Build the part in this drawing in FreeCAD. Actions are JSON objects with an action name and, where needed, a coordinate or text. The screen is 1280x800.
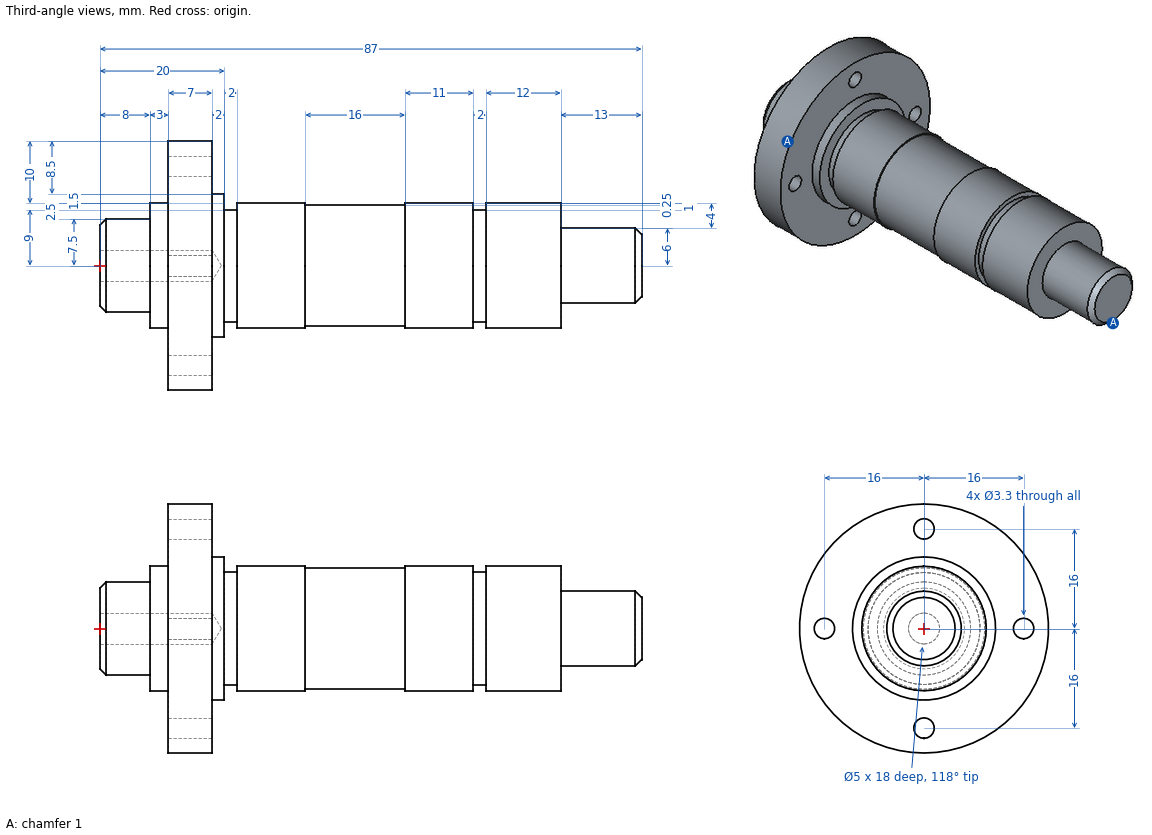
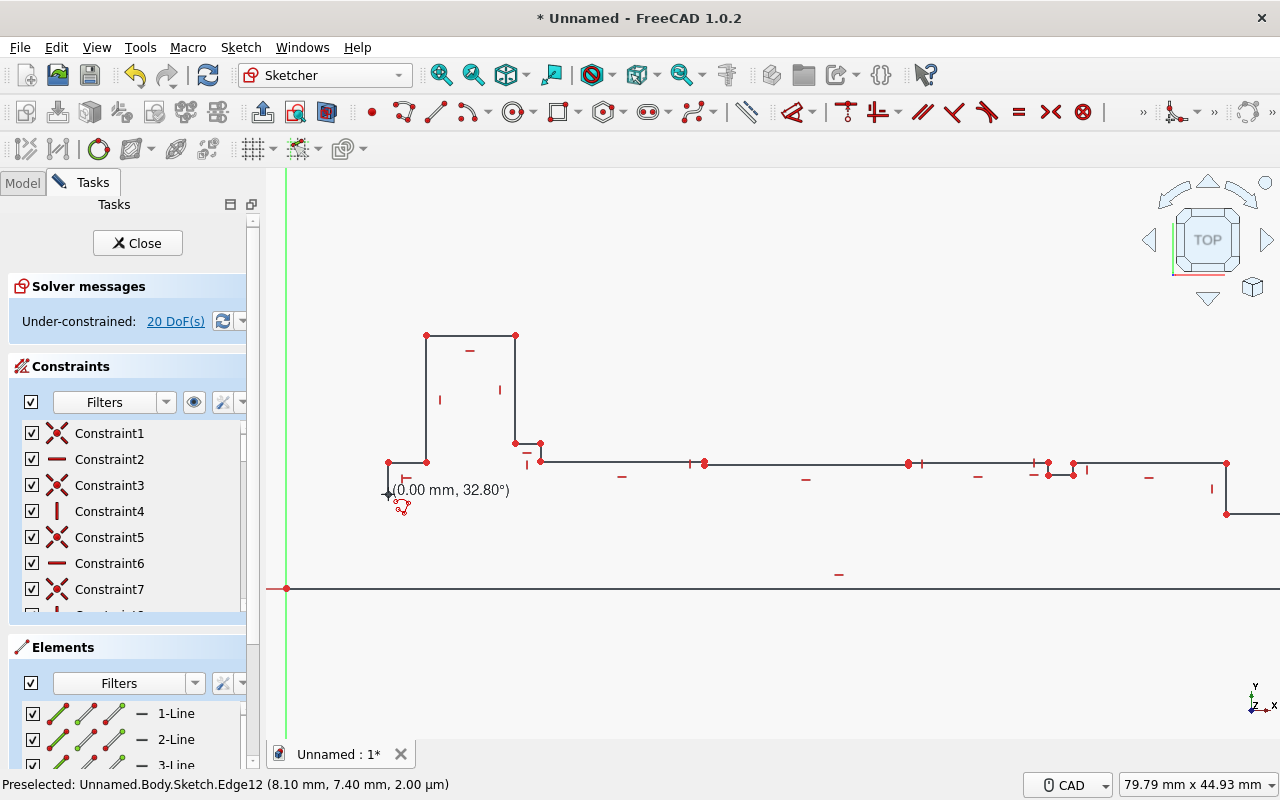
{"action": "scroll", "coordinate": [541, 443], "scroll_direction": "down", "scroll_amount": 3}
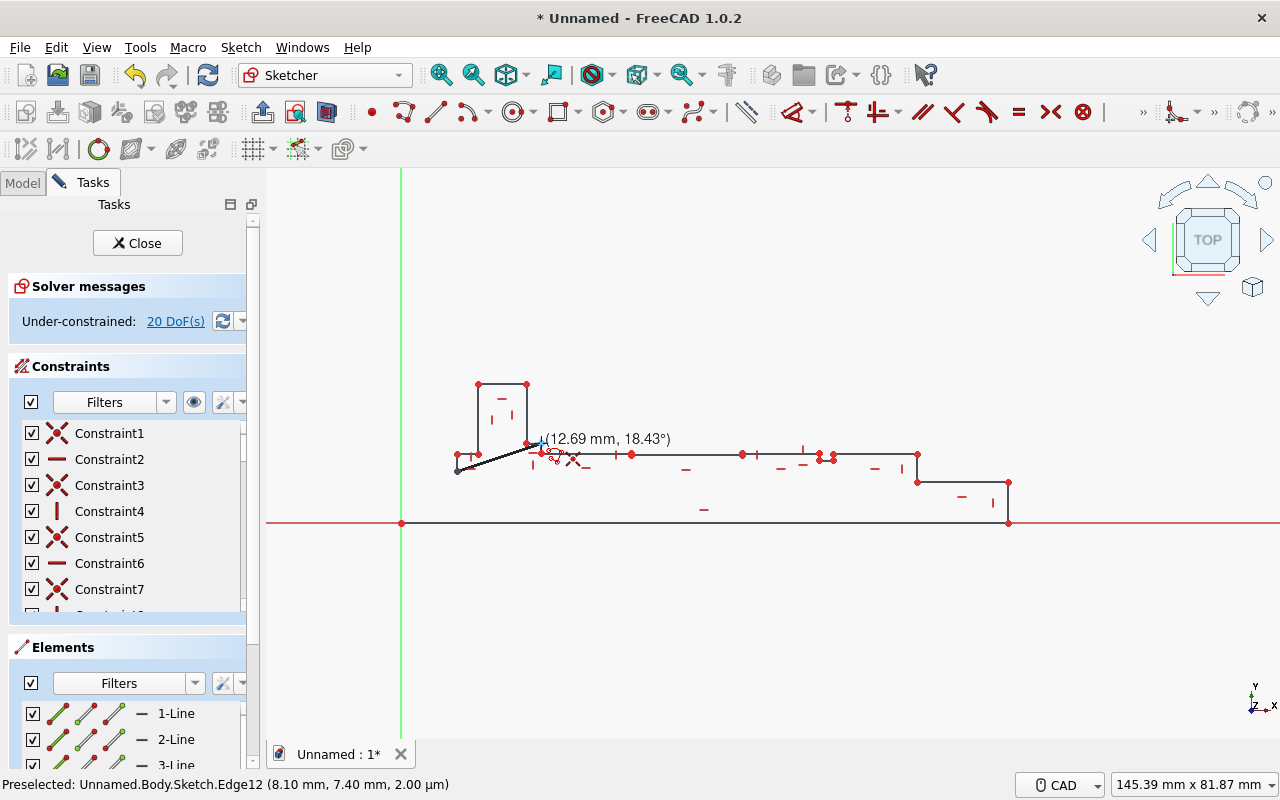
{"action": "left_click", "coordinate": [410, 471]}
{"action": "left_click", "coordinate": [401, 523]}
{"action": "key", "text": "Escape"}
{"action": "key", "text": "Escape"}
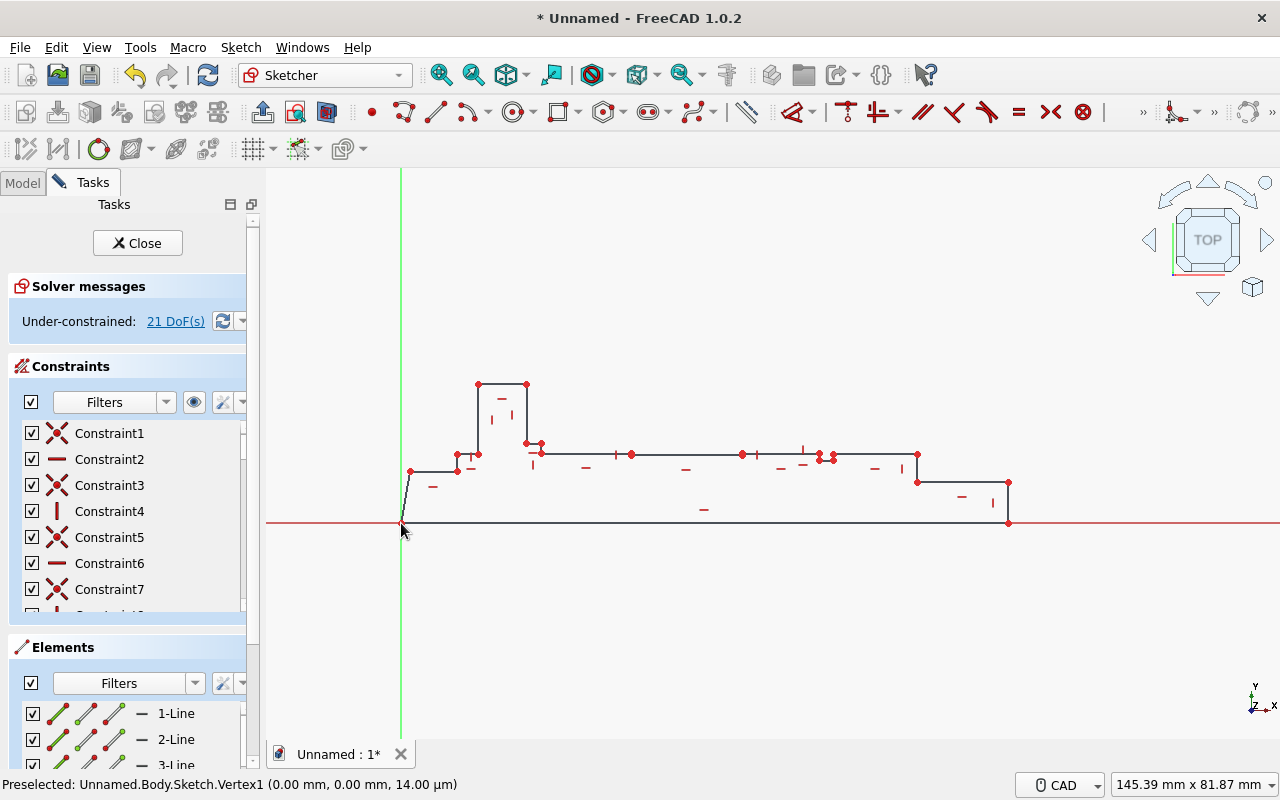
{"action": "left_click", "coordinate": [404, 508]}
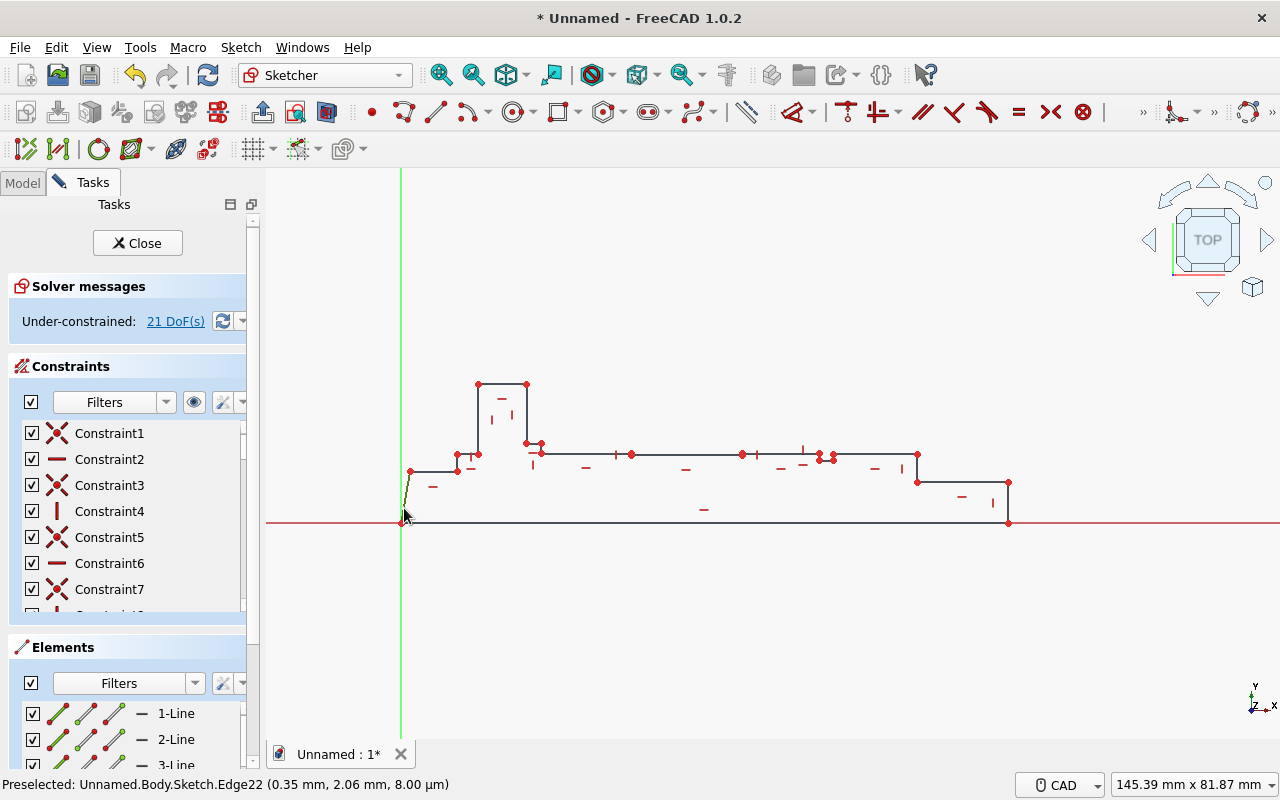
{"action": "left_click", "coordinate": [900, 112]}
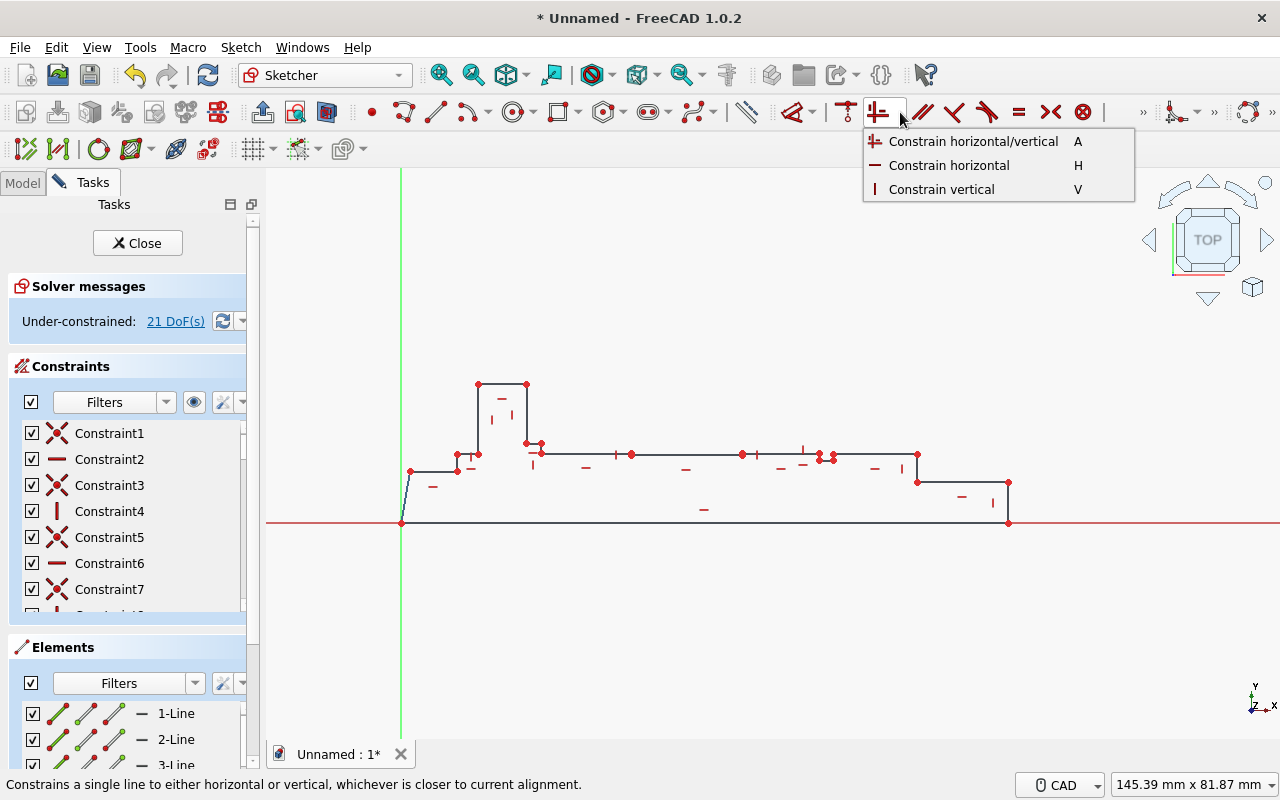
{"action": "left_click", "coordinate": [999, 189]}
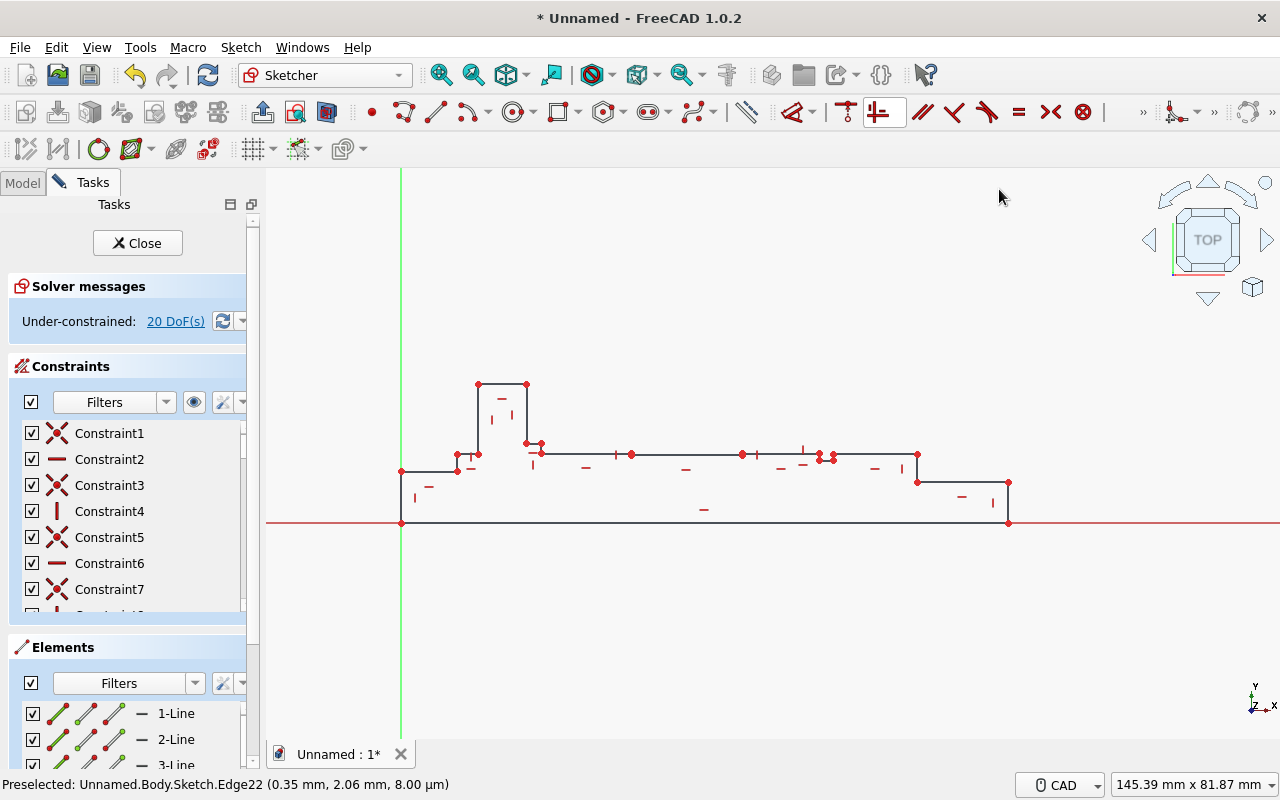
{"action": "left_click", "coordinate": [1008, 511]}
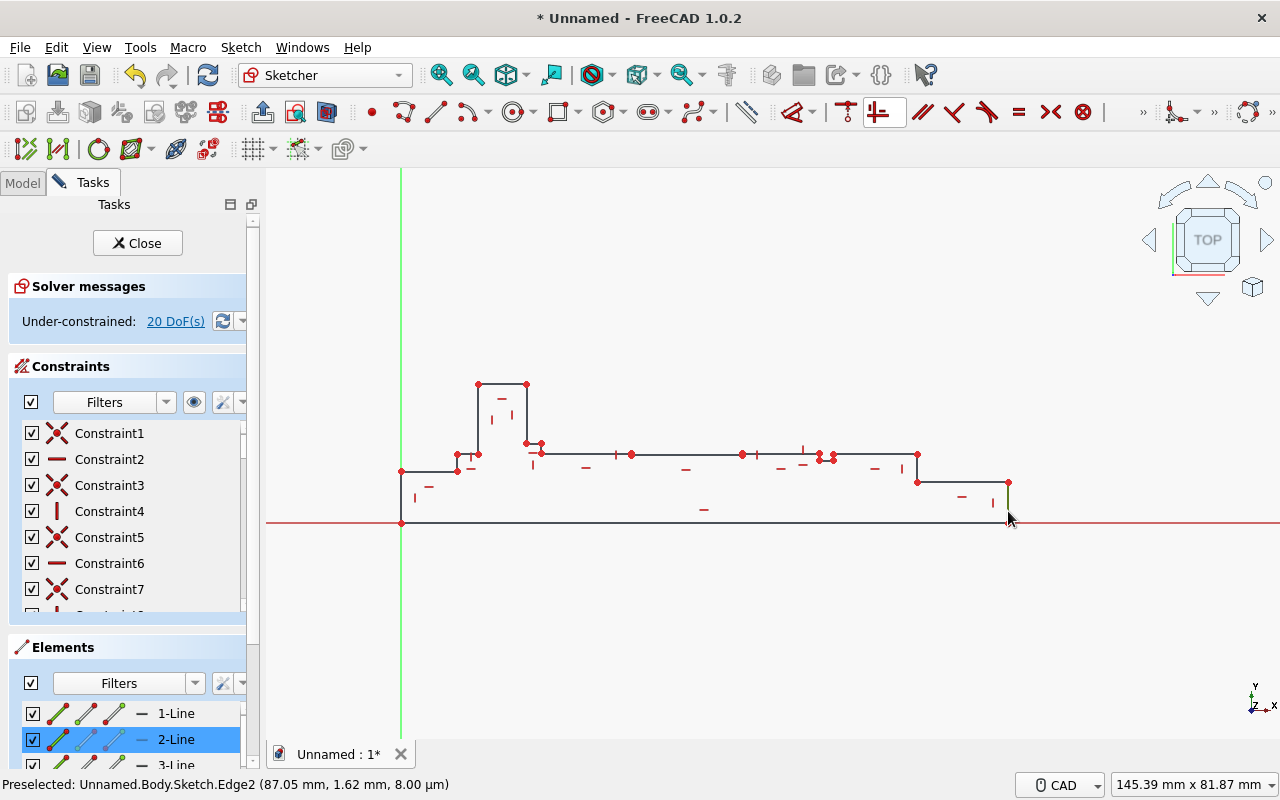
{"action": "left_click", "coordinate": [814, 112]}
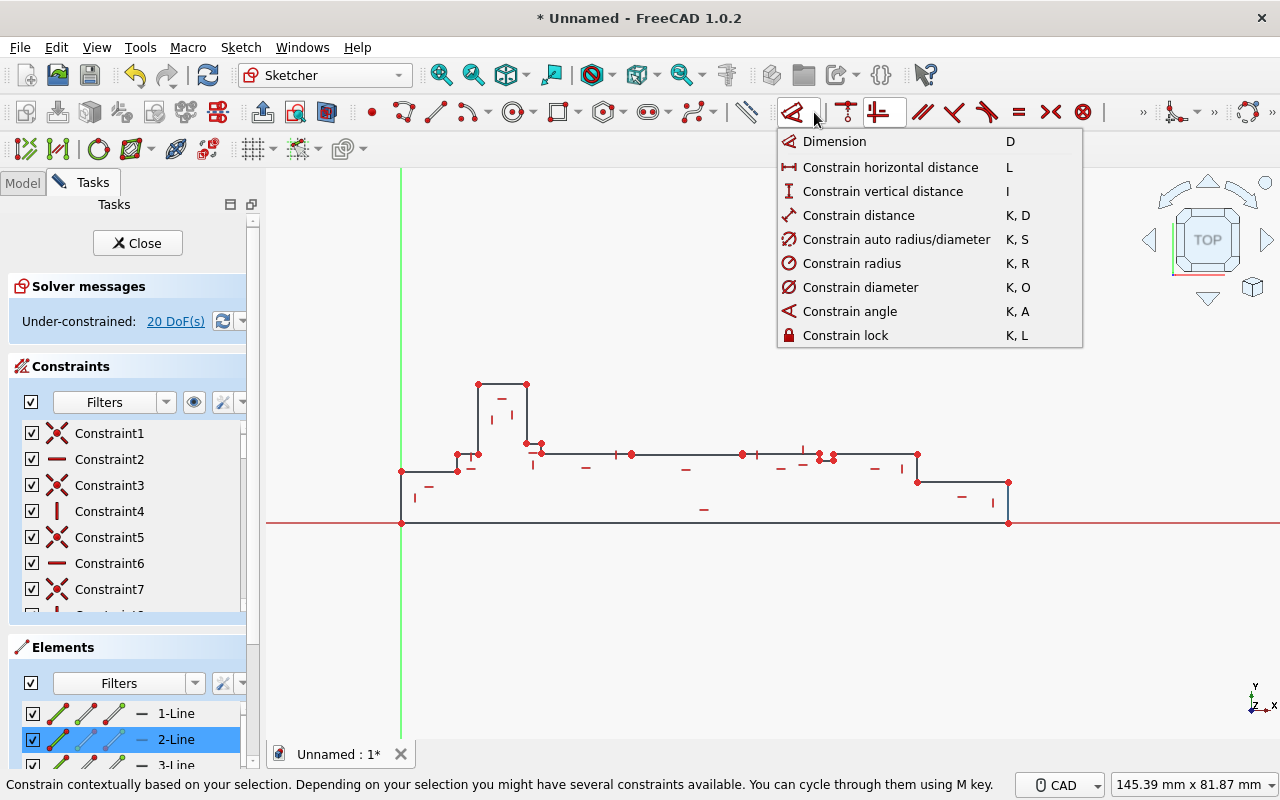
{"action": "left_click", "coordinate": [930, 191]}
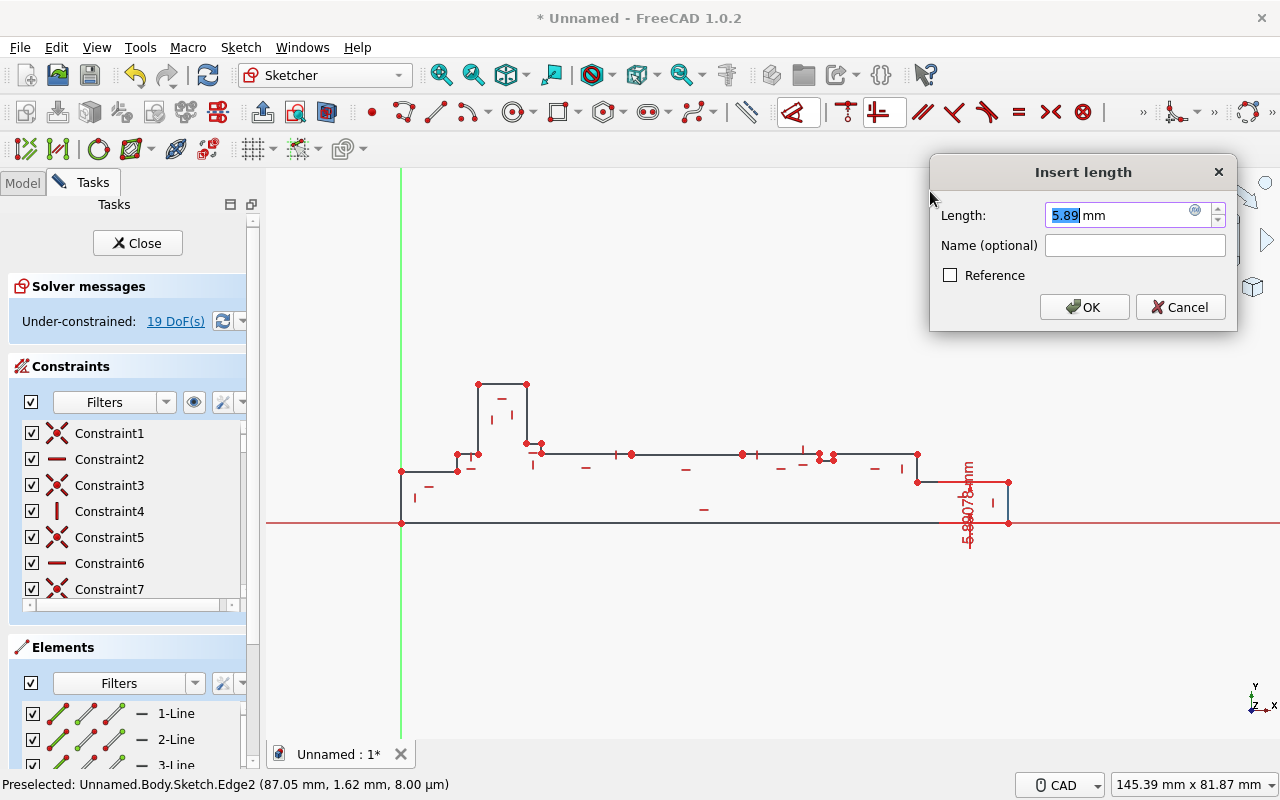
{"action": "type", "text": "6"}
{"action": "key", "text": "Return"}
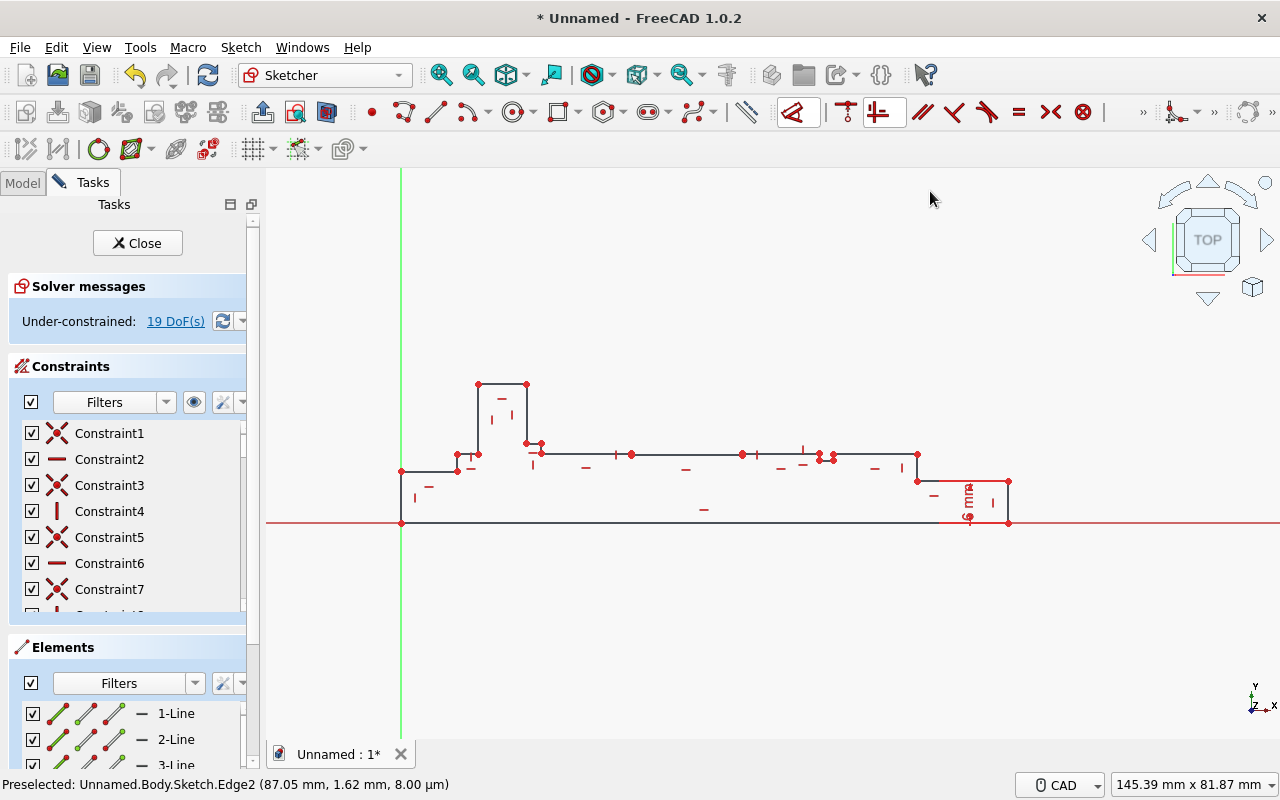
{"action": "scroll", "coordinate": [917, 471], "scroll_direction": "up", "scroll_amount": 2}